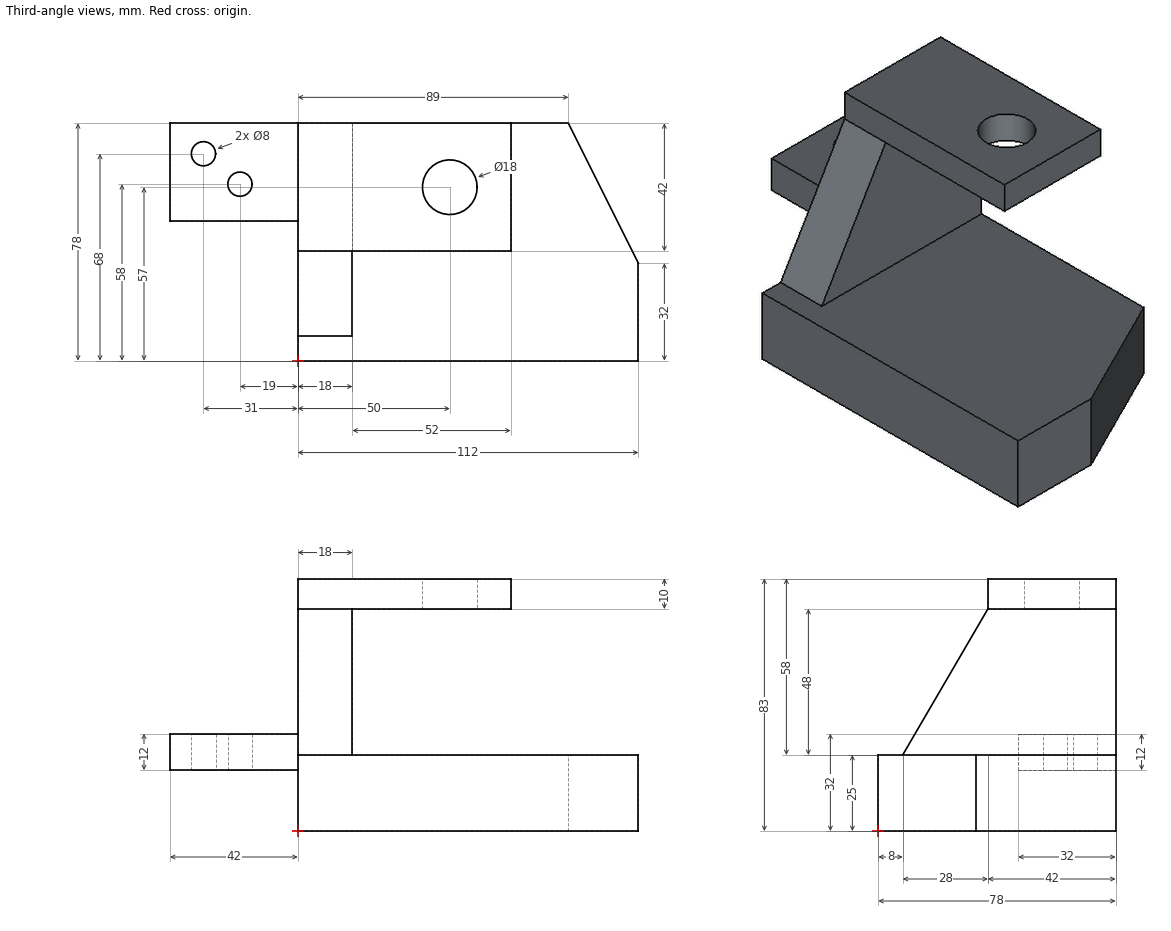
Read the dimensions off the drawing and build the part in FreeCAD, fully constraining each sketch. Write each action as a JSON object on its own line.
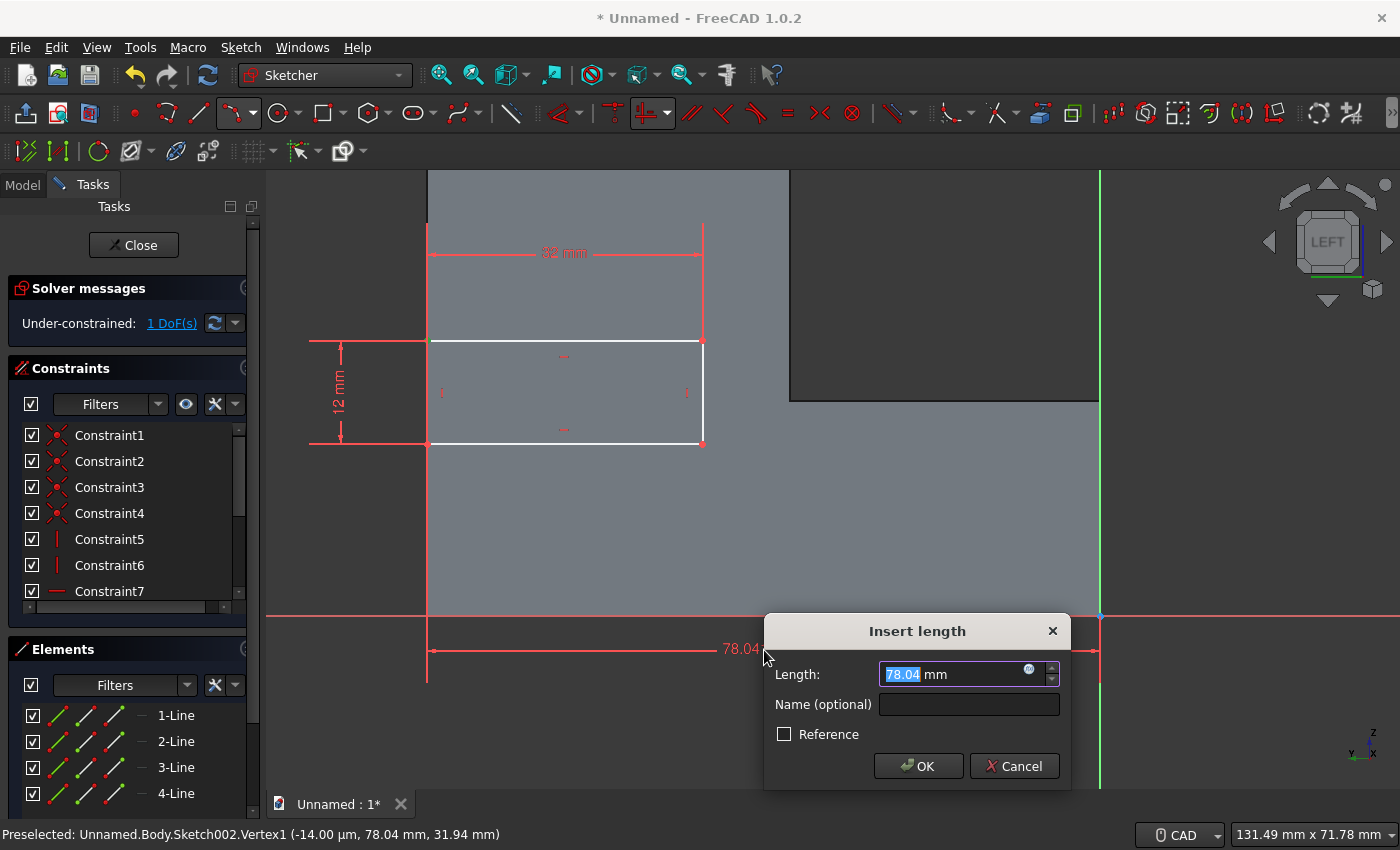
{"action": "type", "text": "78"}
{"action": "key", "text": "Return"}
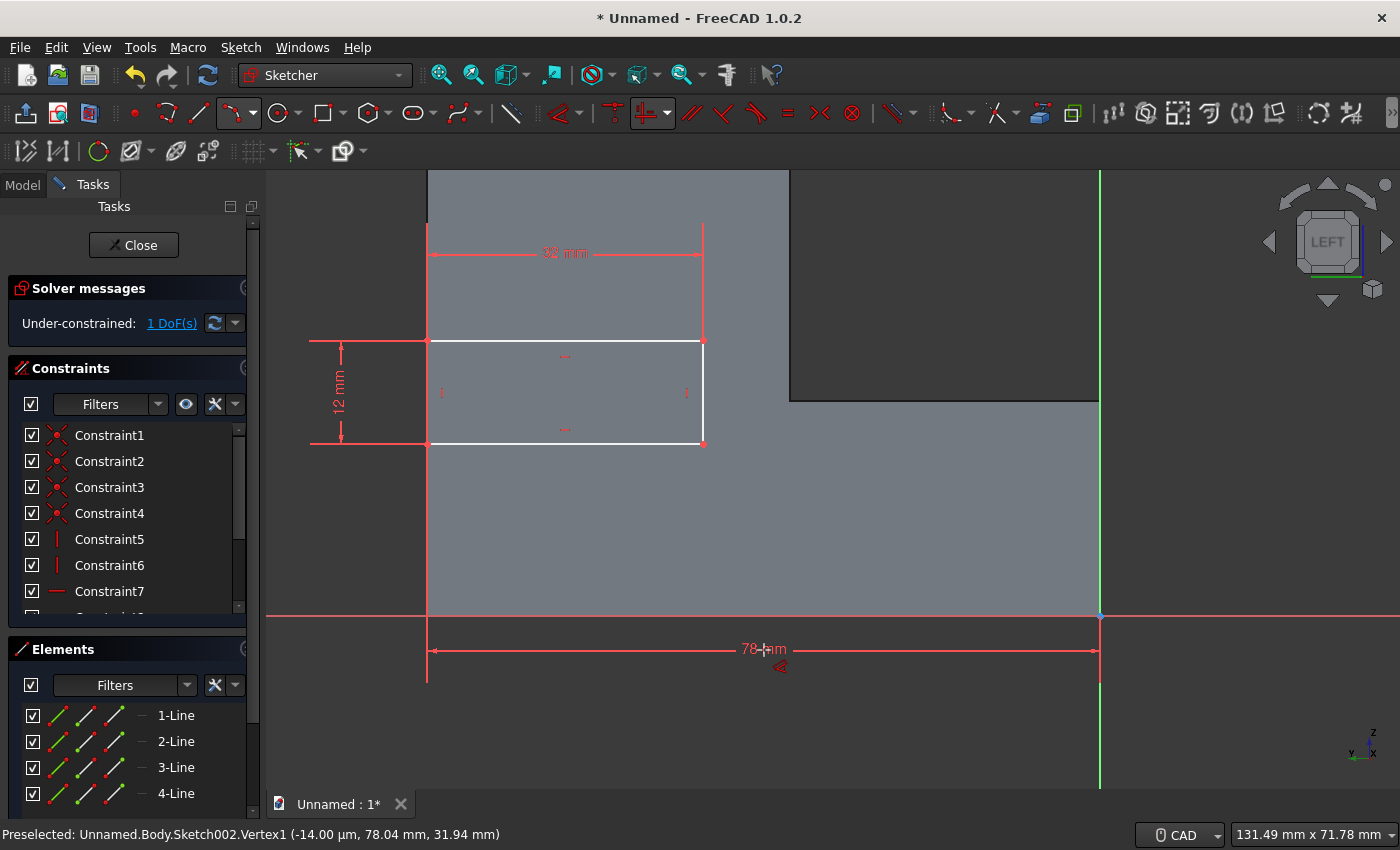
{"action": "left_click", "coordinate": [427, 341]}
{"action": "left_click", "coordinate": [1134, 479]}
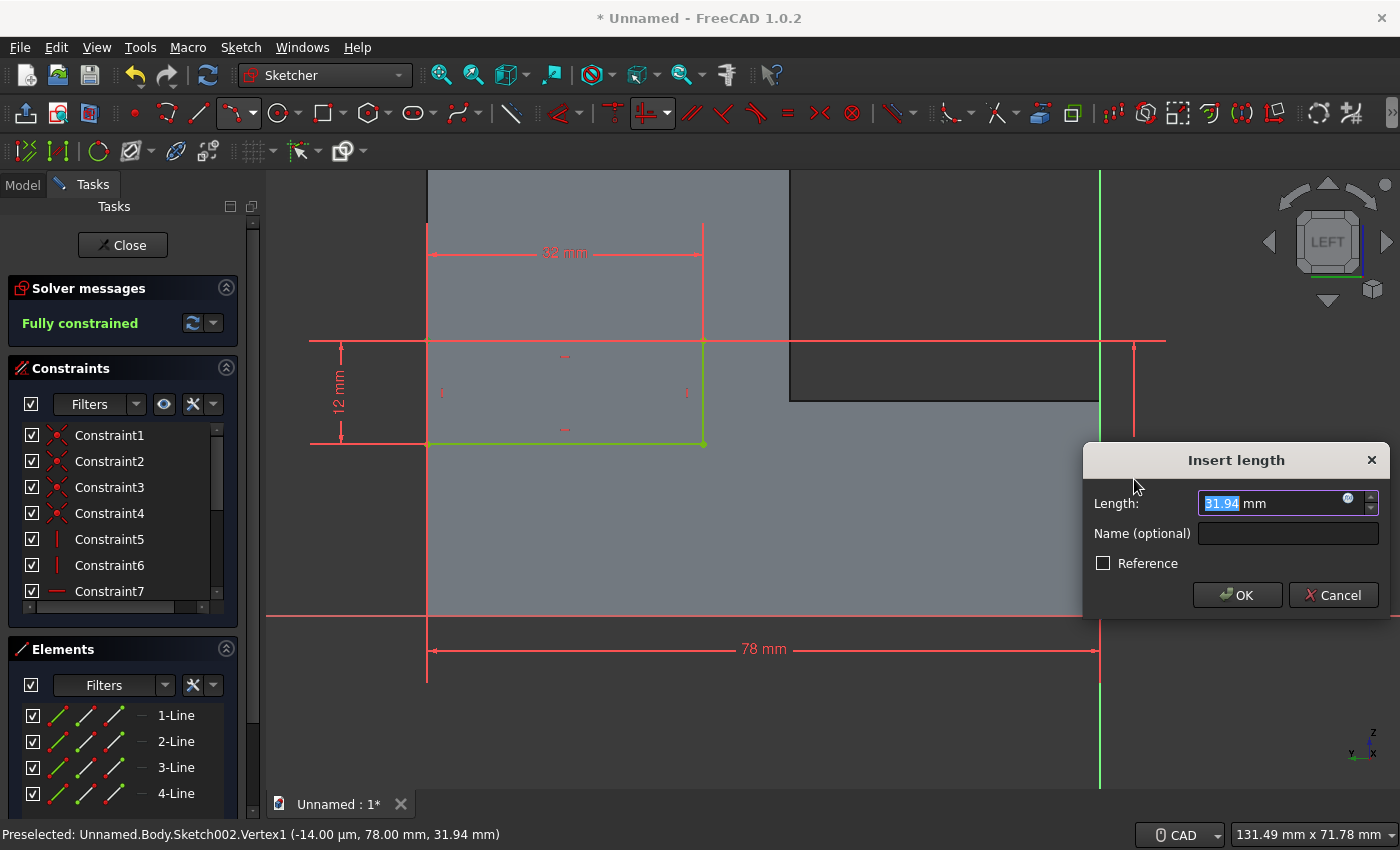
{"action": "type", "text": "32"}
{"action": "key", "text": "Return"}
{"action": "key", "text": "Escape"}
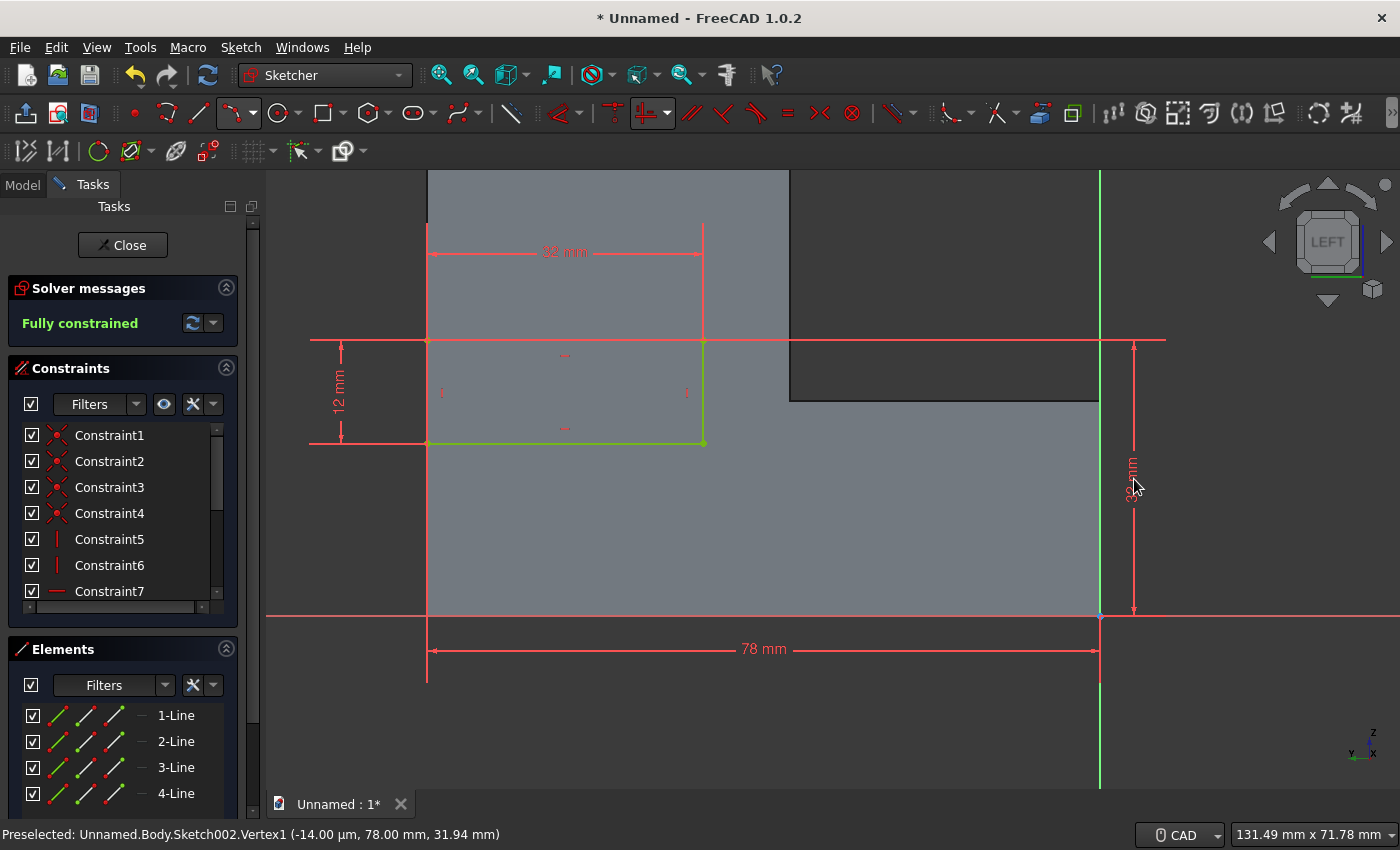
{"action": "left_click", "coordinate": [123, 245]}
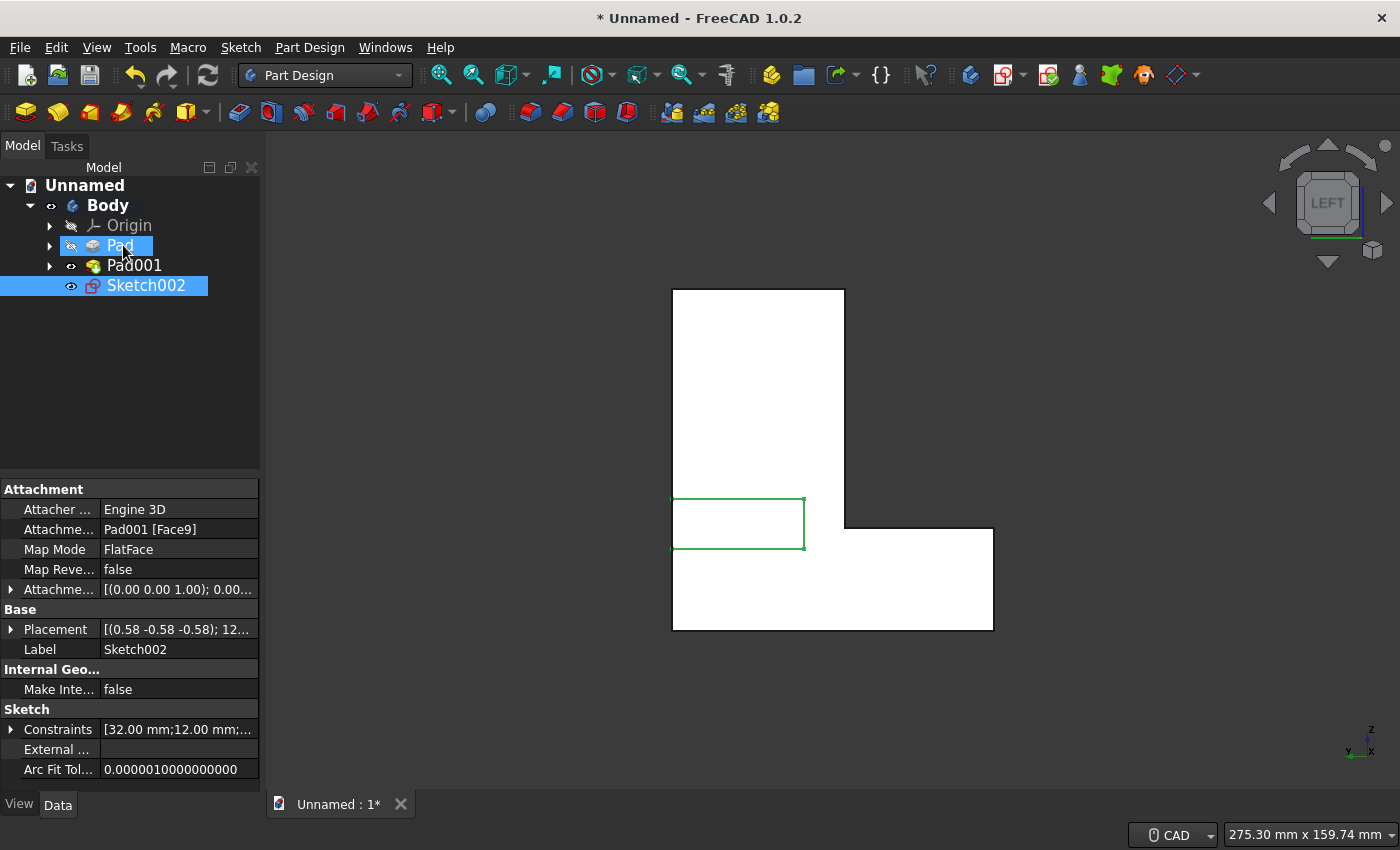
{"action": "left_click", "coordinate": [26, 112]}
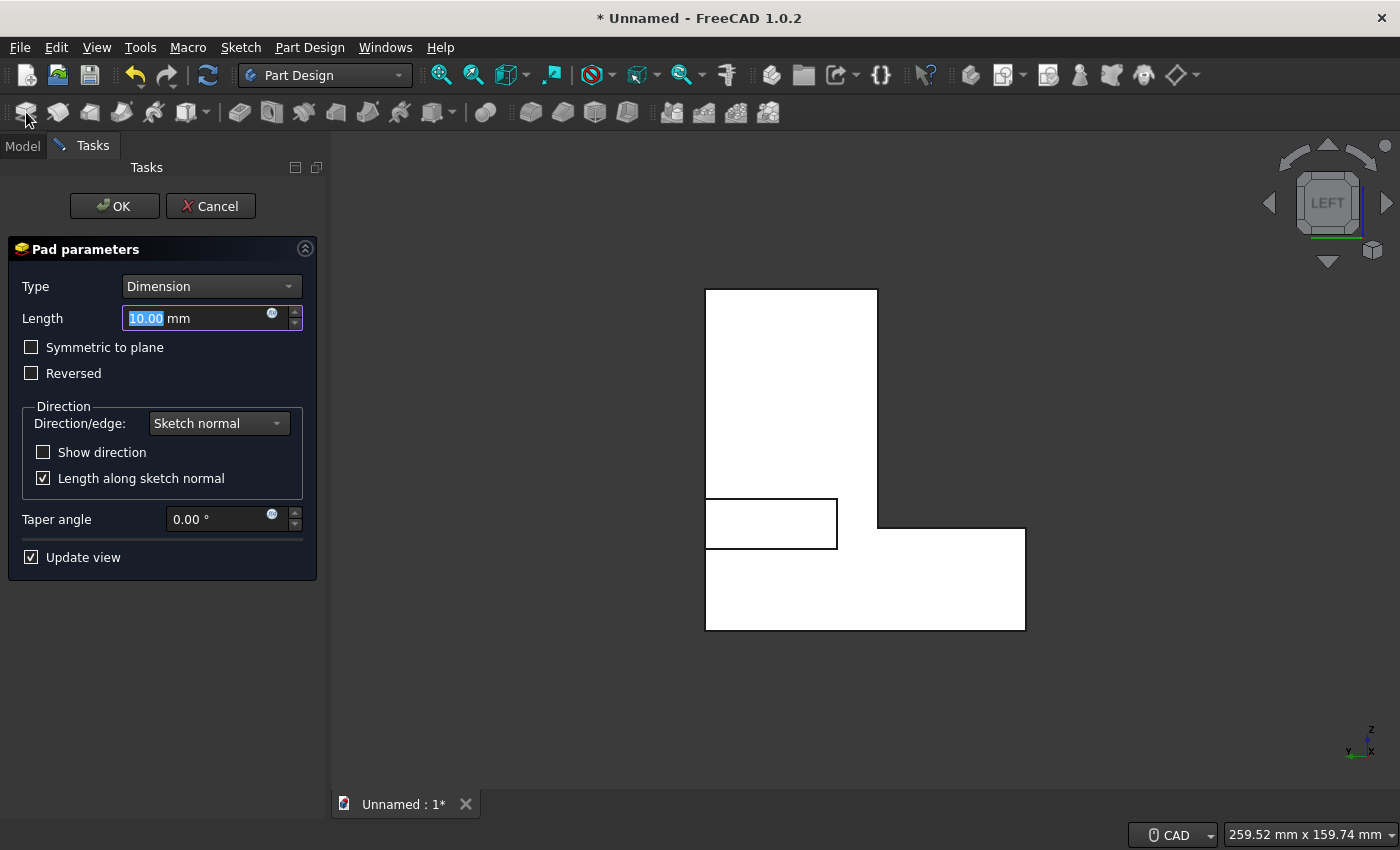
{"action": "type", "text": "42"}
{"action": "key", "text": "Tab"}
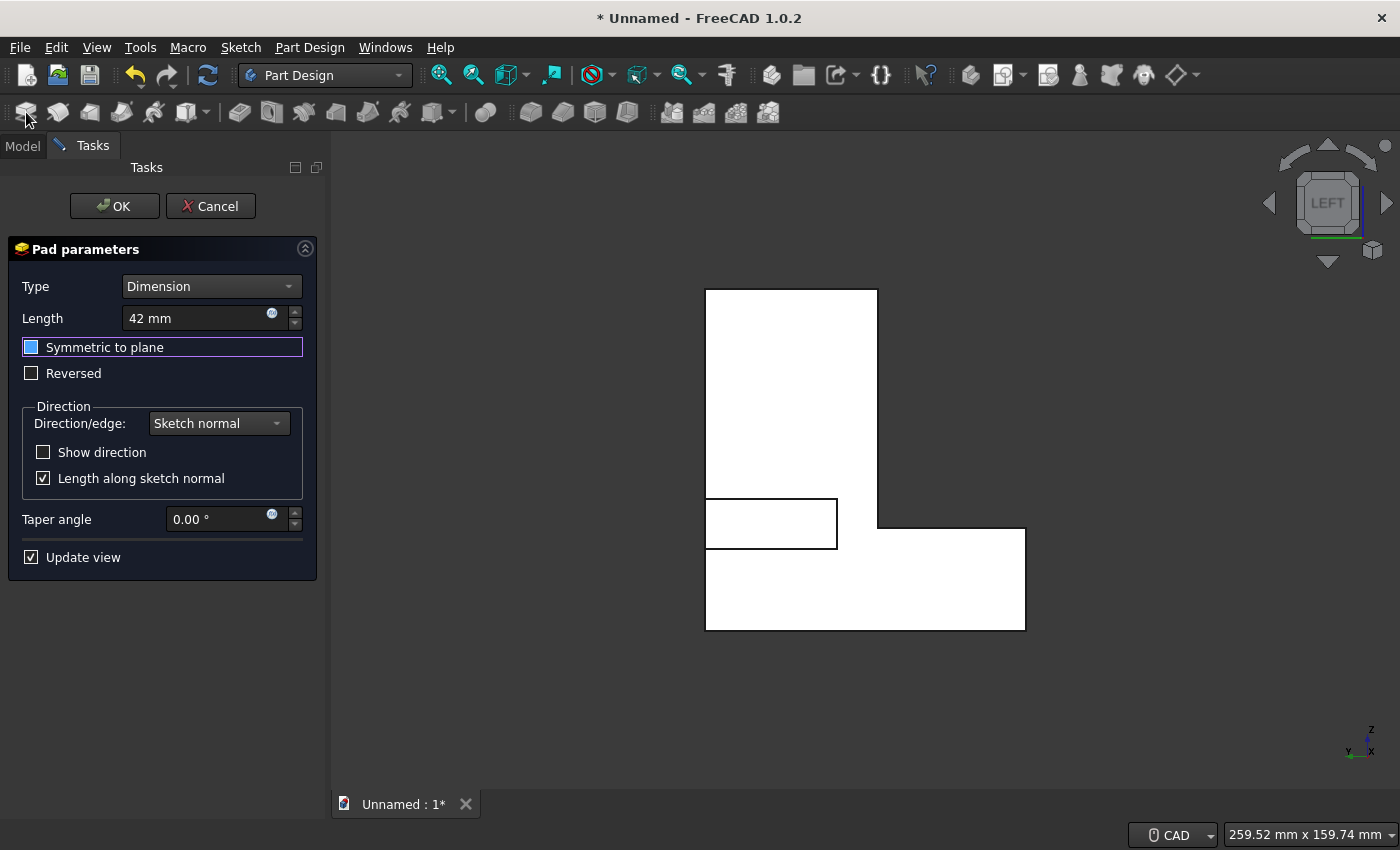
{"action": "left_click", "coordinate": [115, 206]}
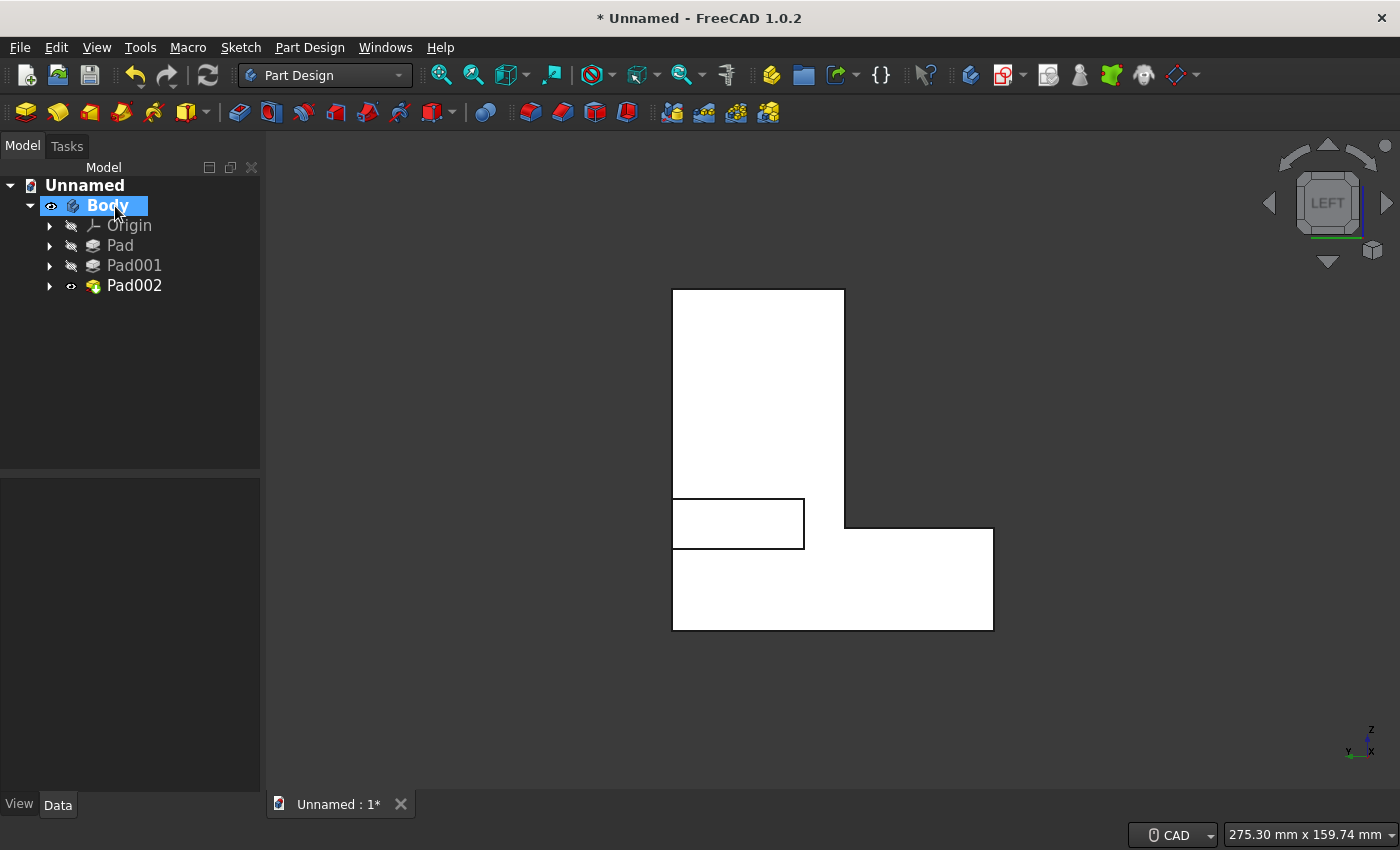
{"action": "key", "text": "0"}